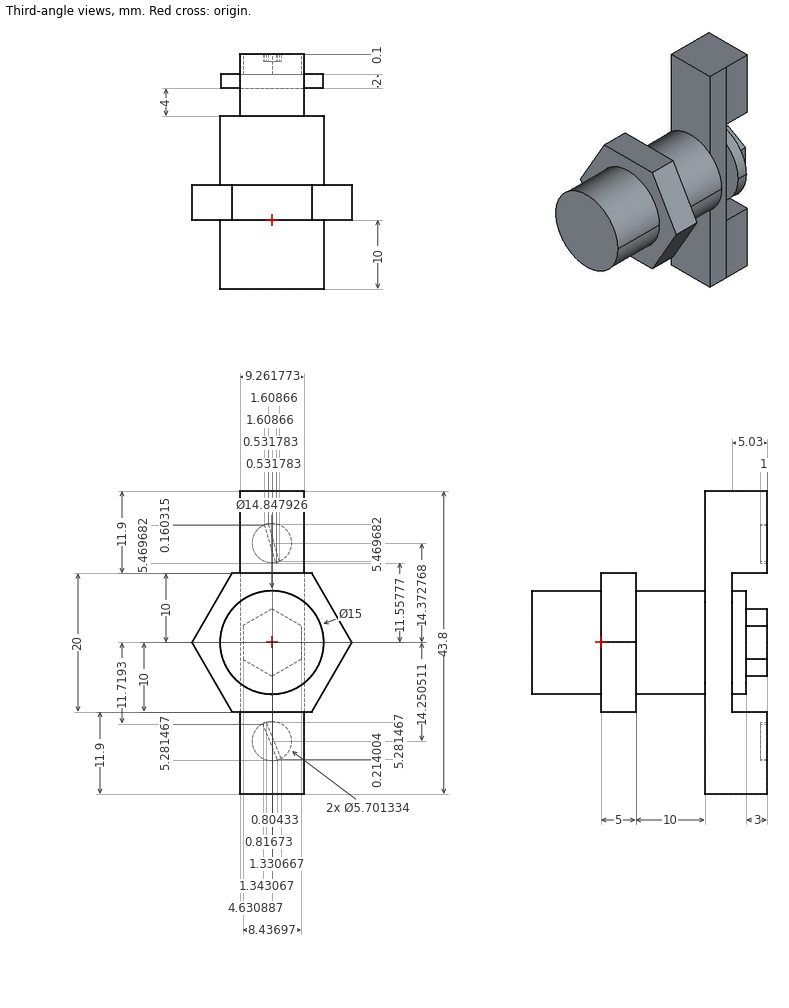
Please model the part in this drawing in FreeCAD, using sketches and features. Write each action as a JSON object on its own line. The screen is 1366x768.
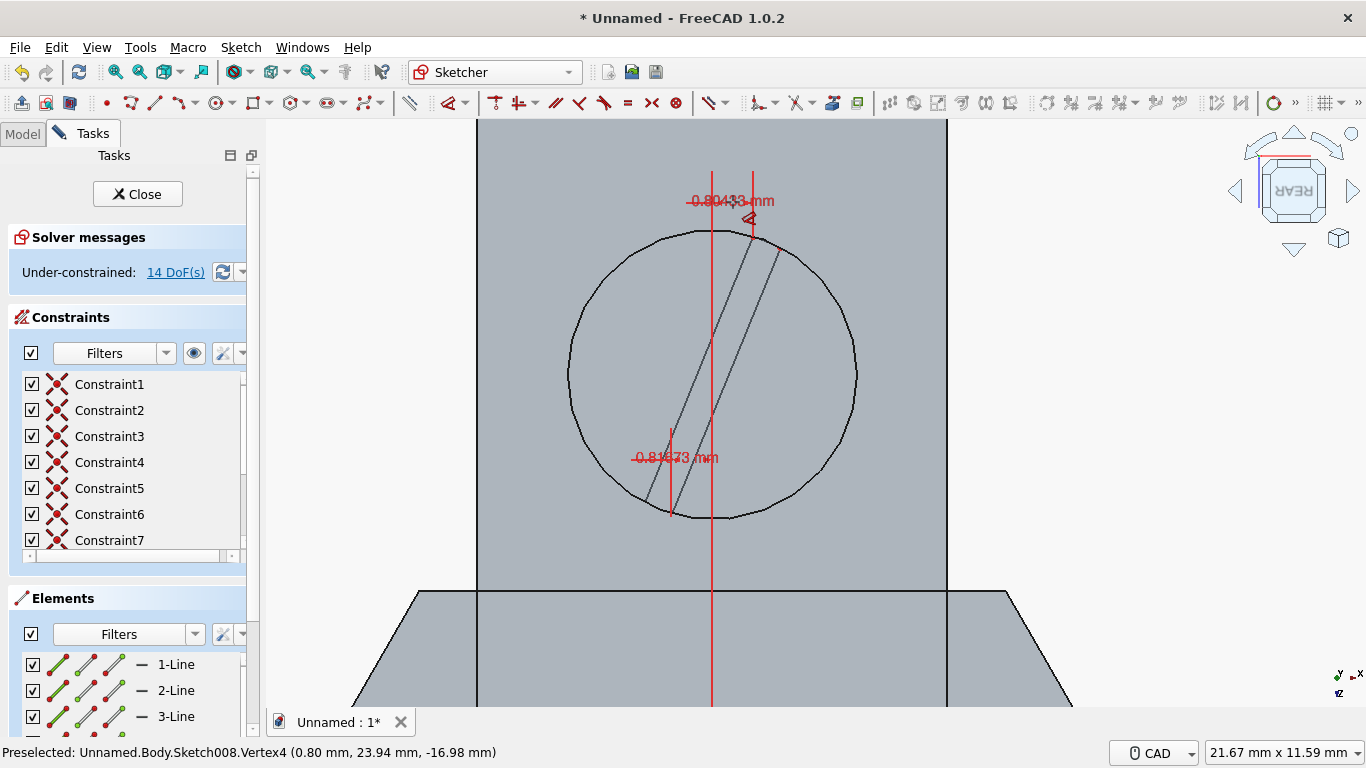
{"action": "left_click", "coordinate": [644, 505]}
{"action": "left_click", "coordinate": [610, 592]}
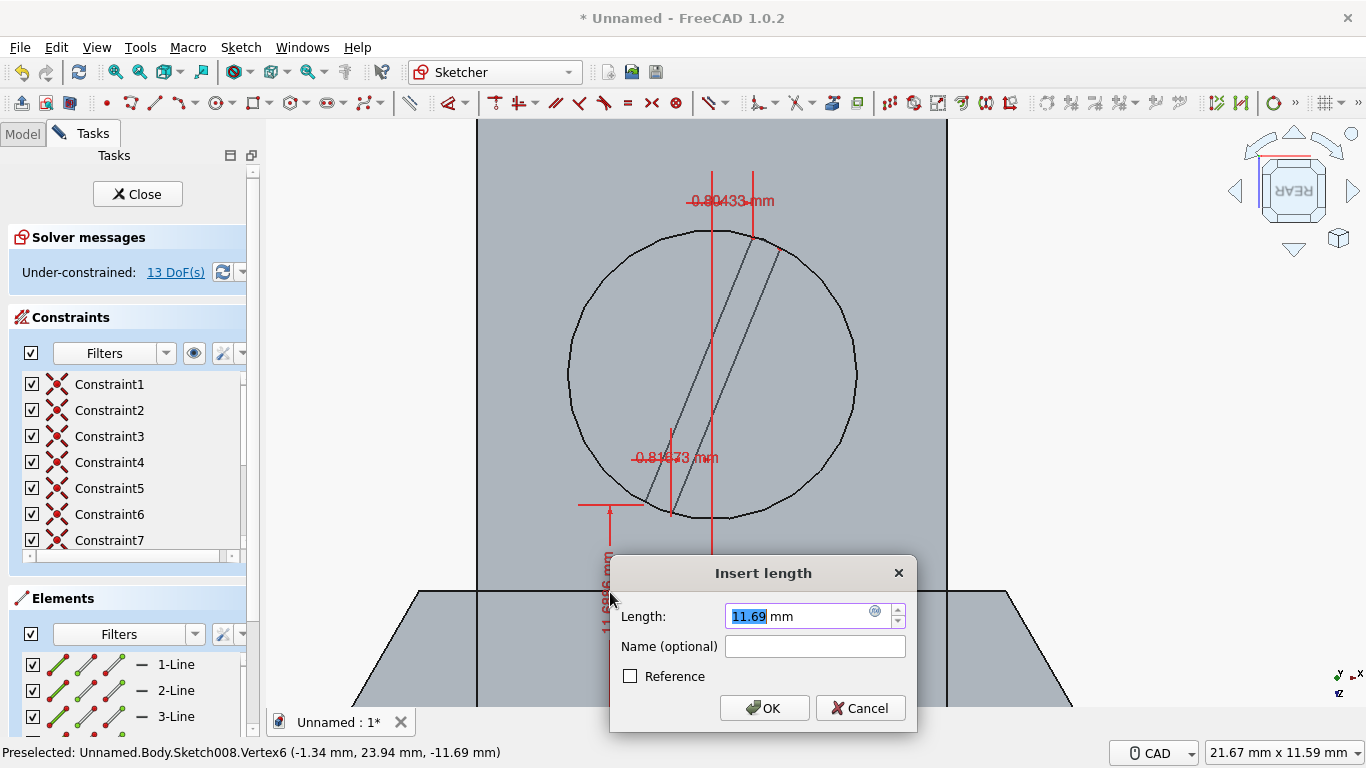
{"action": "type", "text": "11.7193"}
{"action": "key", "text": "Return"}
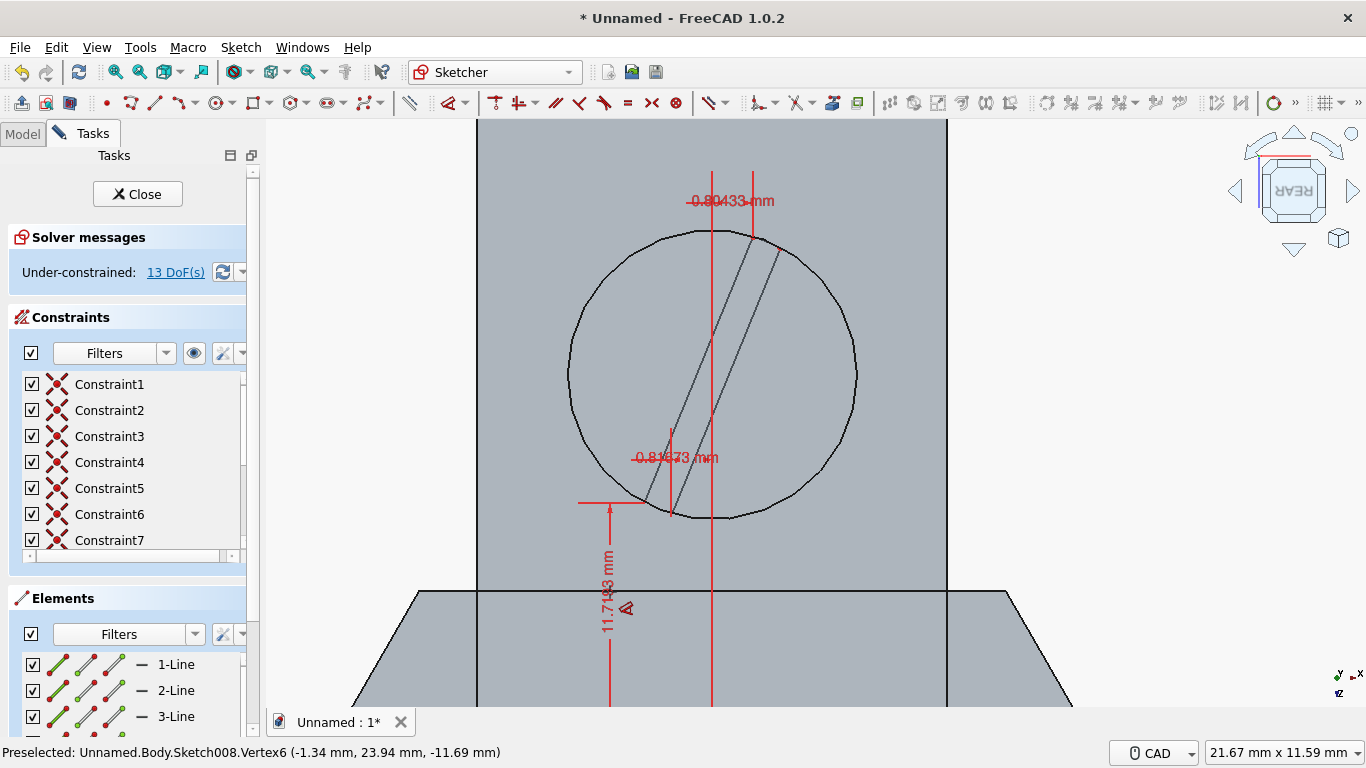
{"action": "scroll", "coordinate": [756, 238], "scroll_direction": "down", "scroll_amount": 8}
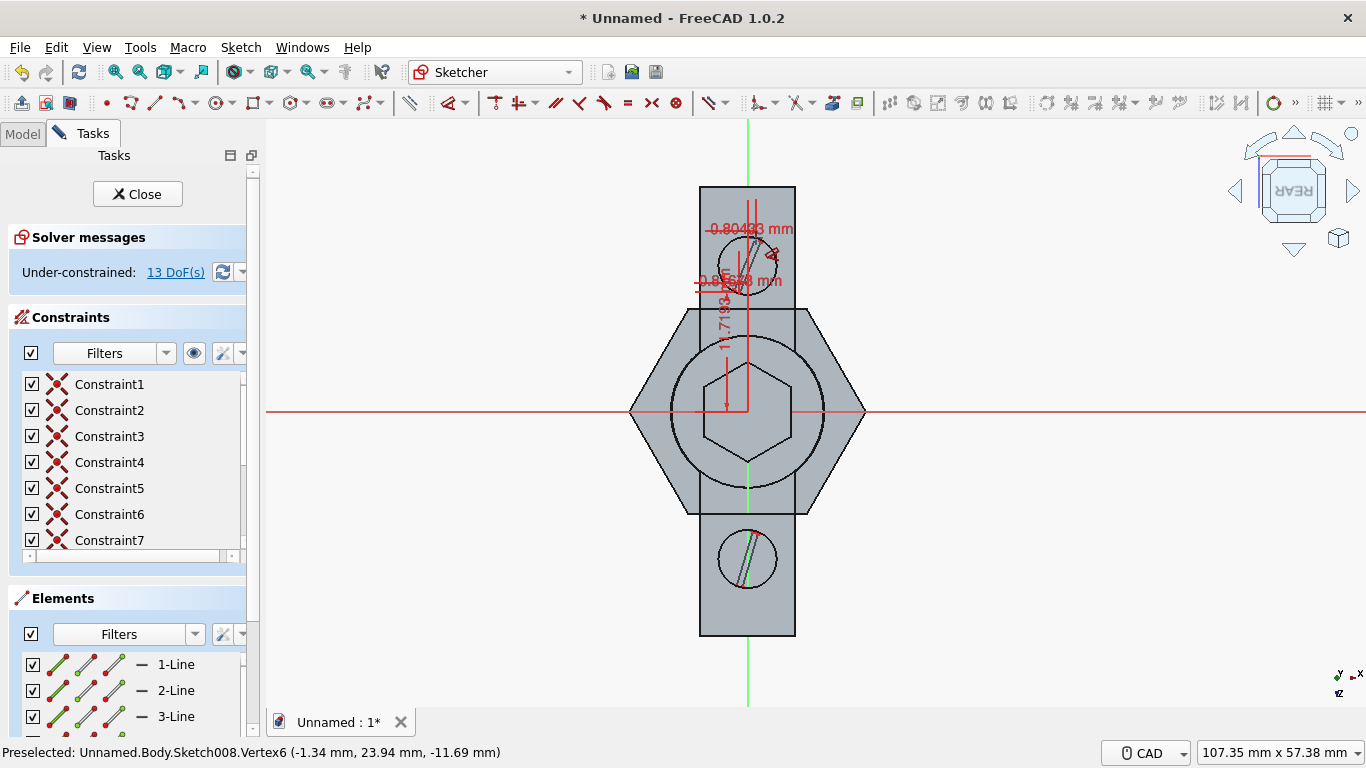
{"action": "scroll", "coordinate": [748, 548], "scroll_direction": "up", "scroll_amount": 5}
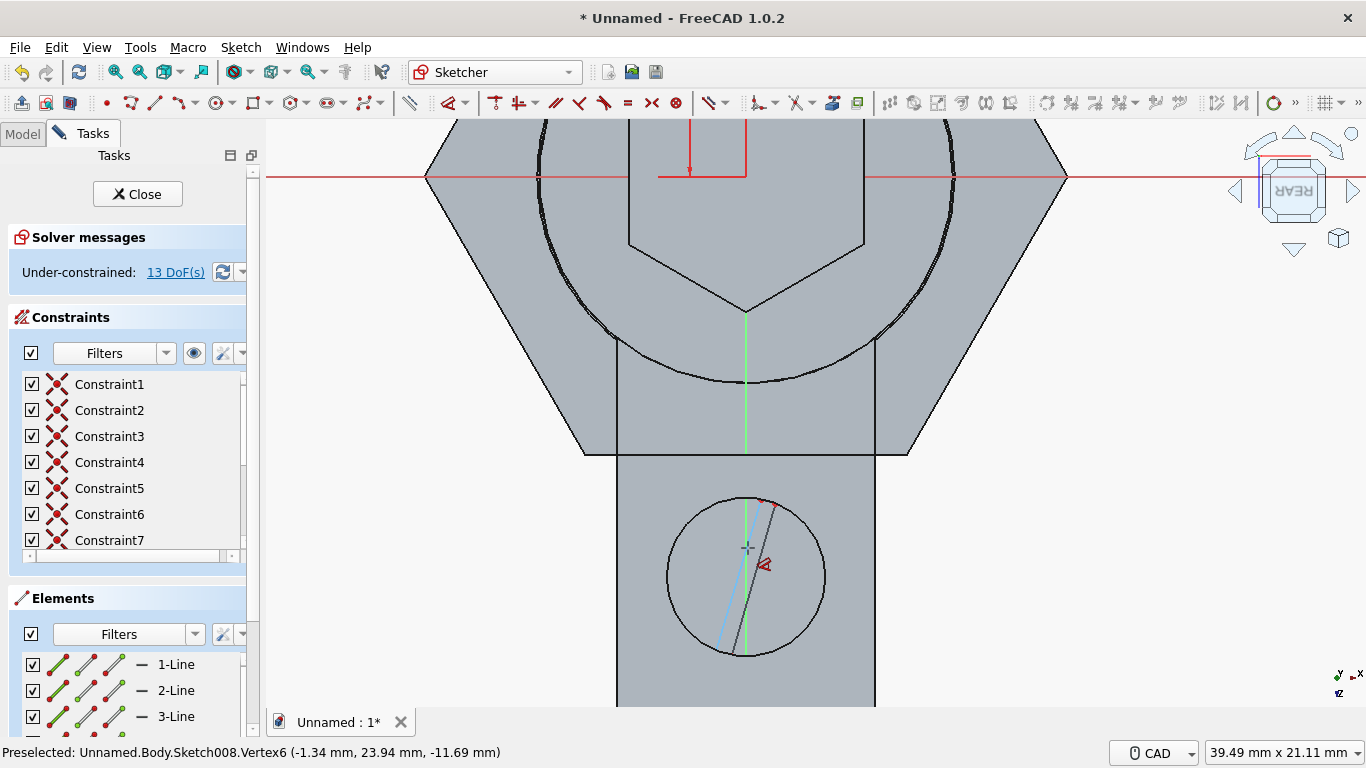
{"action": "left_click", "coordinate": [748, 546]}
{"action": "left_click", "coordinate": [728, 466]}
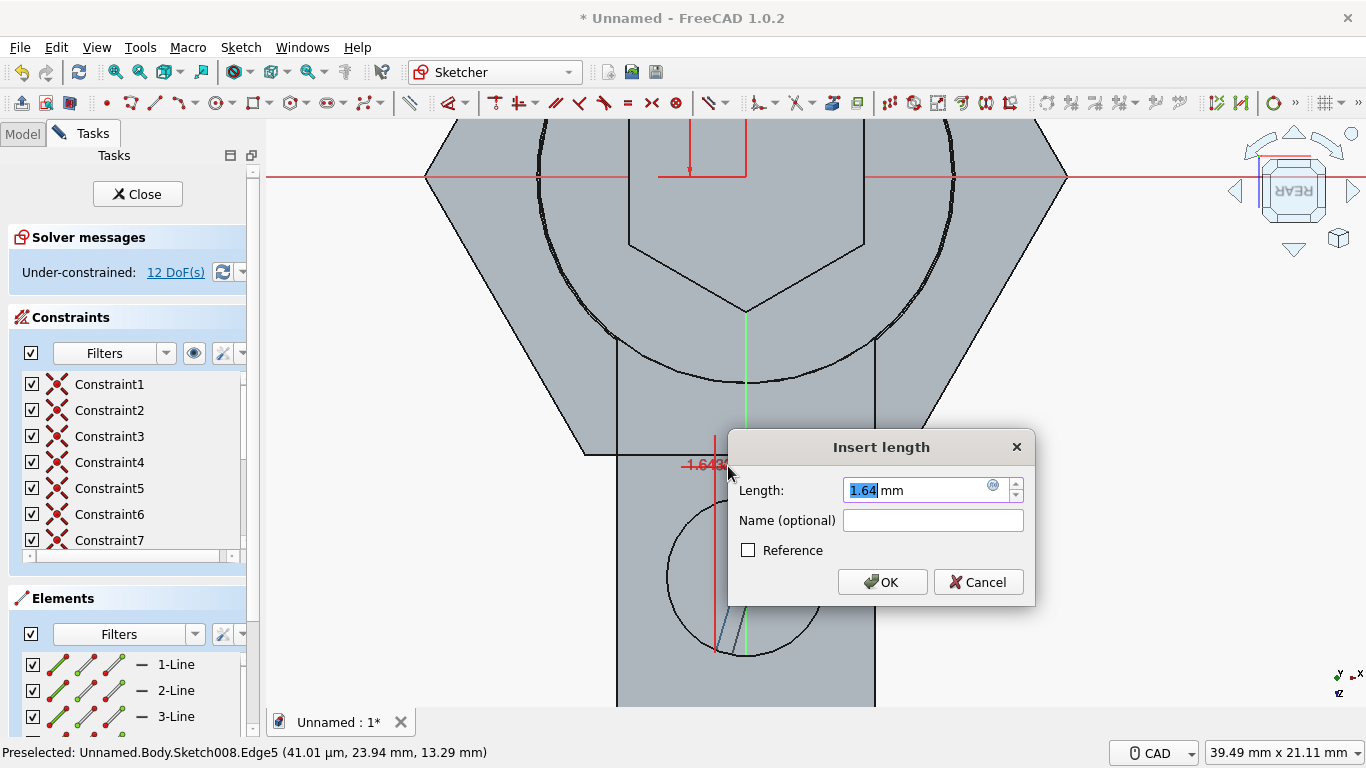
{"action": "type", "text": "1.60866"}
{"action": "key", "text": "Return"}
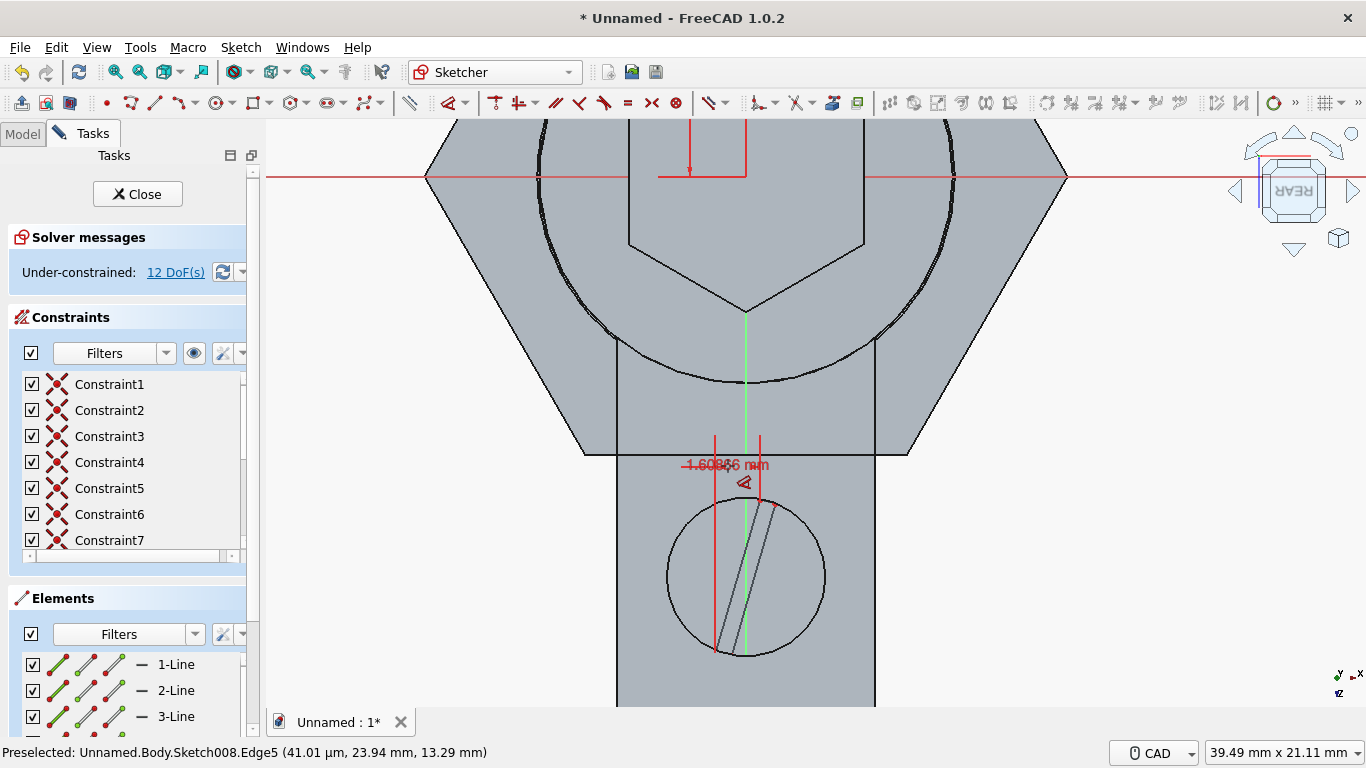
{"action": "left_click", "coordinate": [745, 611]}
{"action": "left_click", "coordinate": [764, 445]}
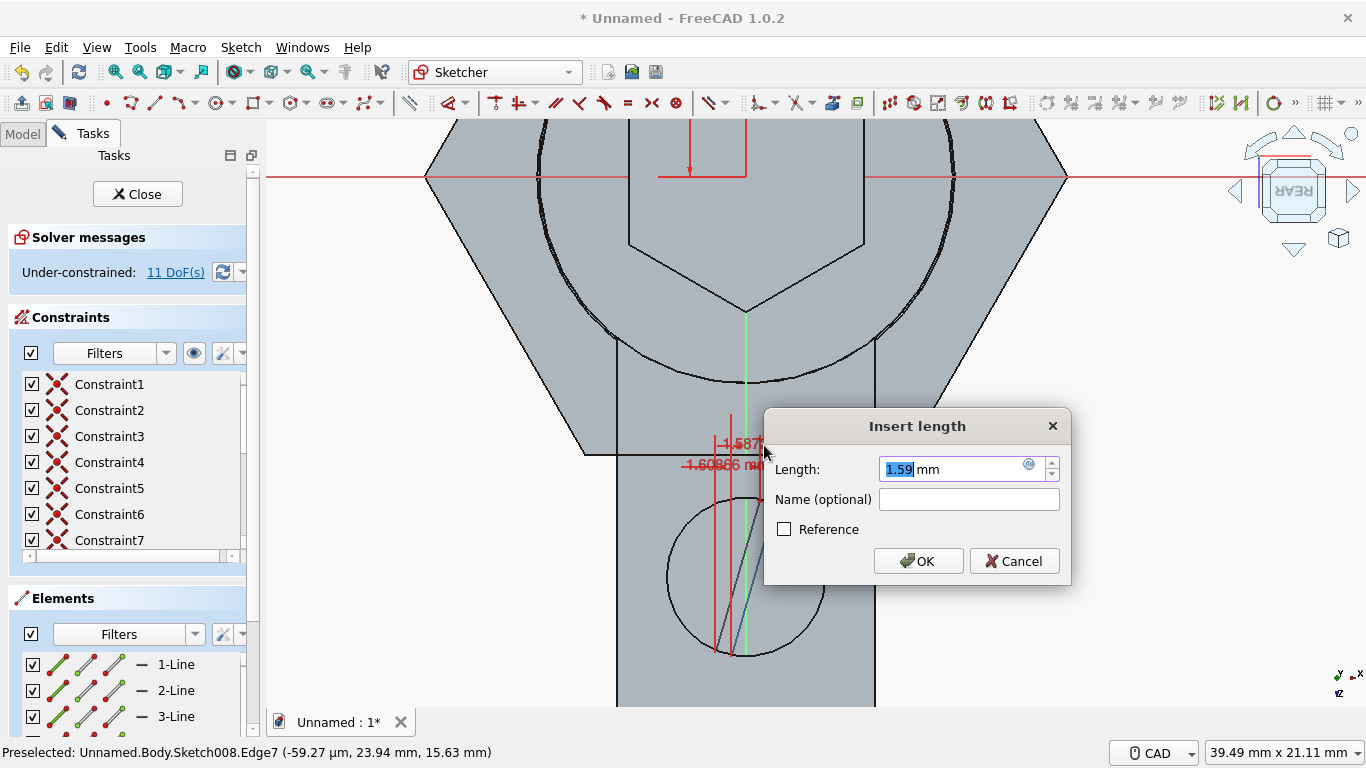
{"action": "type", "text": "1.60866"}
{"action": "key", "text": "Return"}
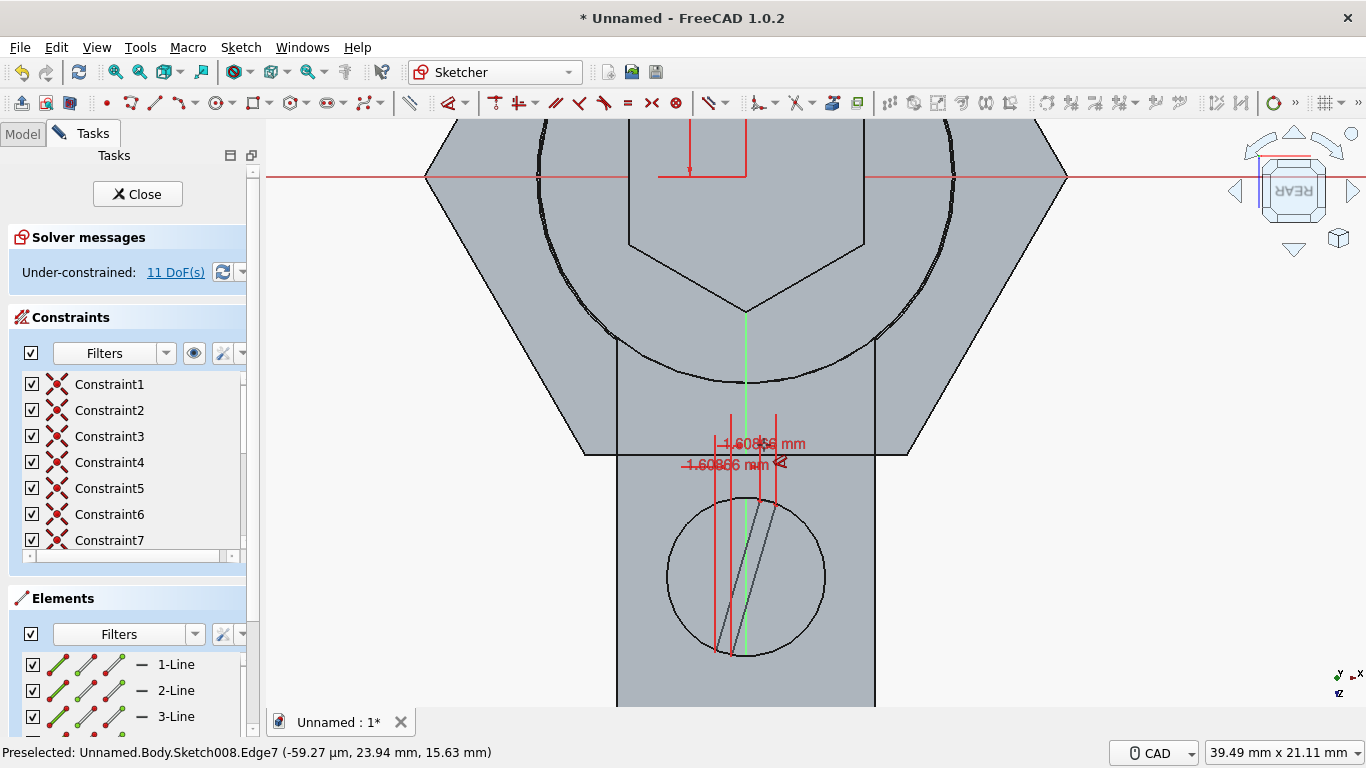
{"action": "scroll", "coordinate": [748, 549], "scroll_direction": "down", "scroll_amount": 5}